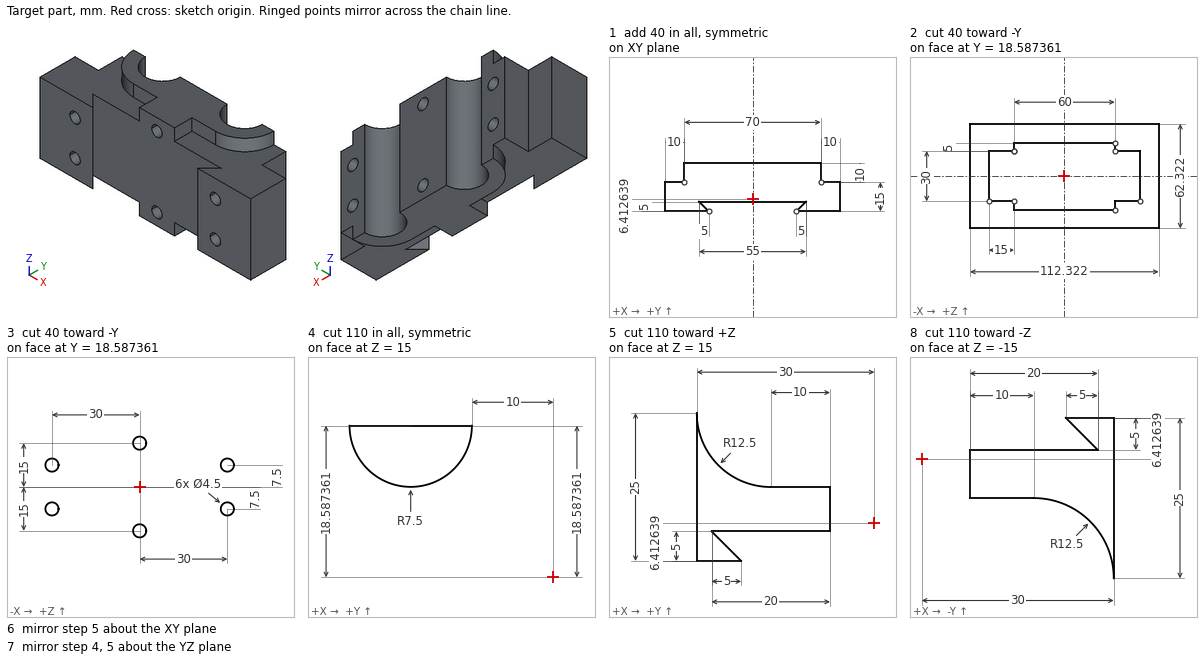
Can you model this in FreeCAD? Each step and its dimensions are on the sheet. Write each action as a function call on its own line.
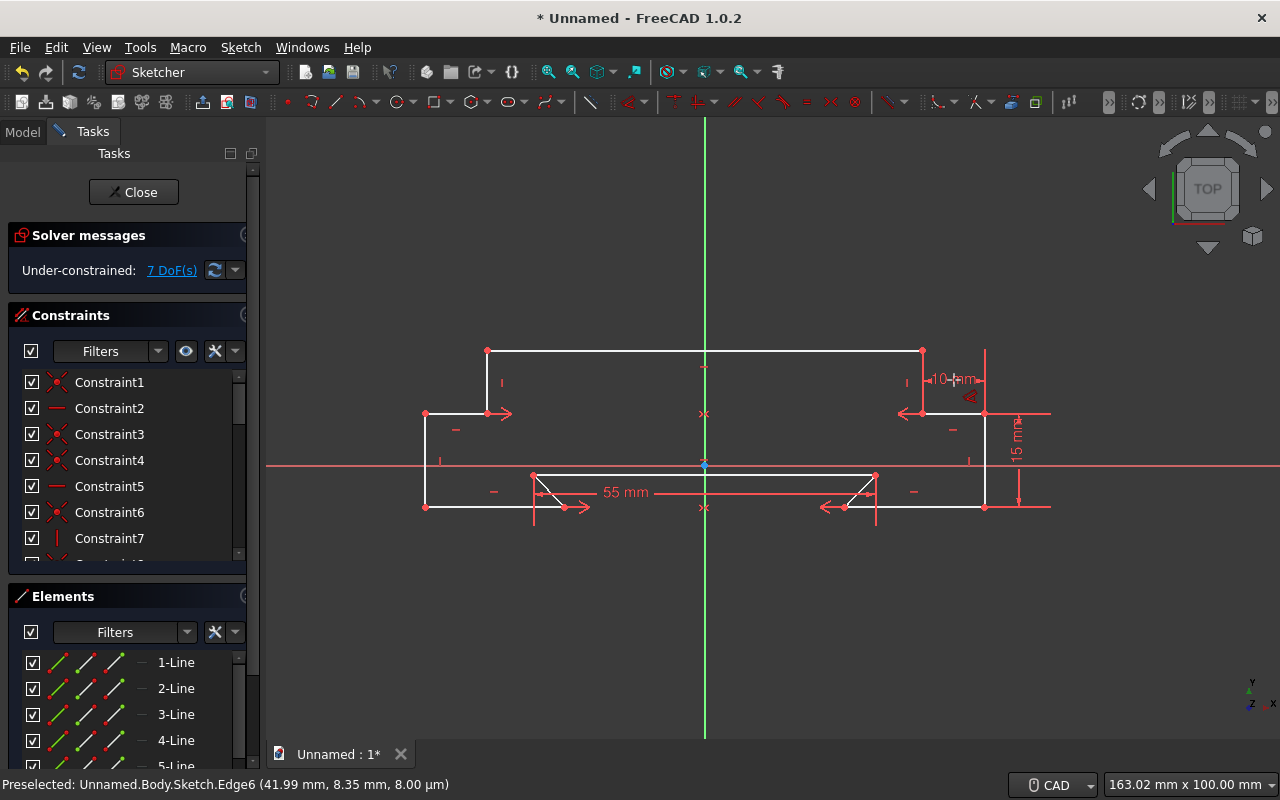
click(923, 395)
click(889, 405)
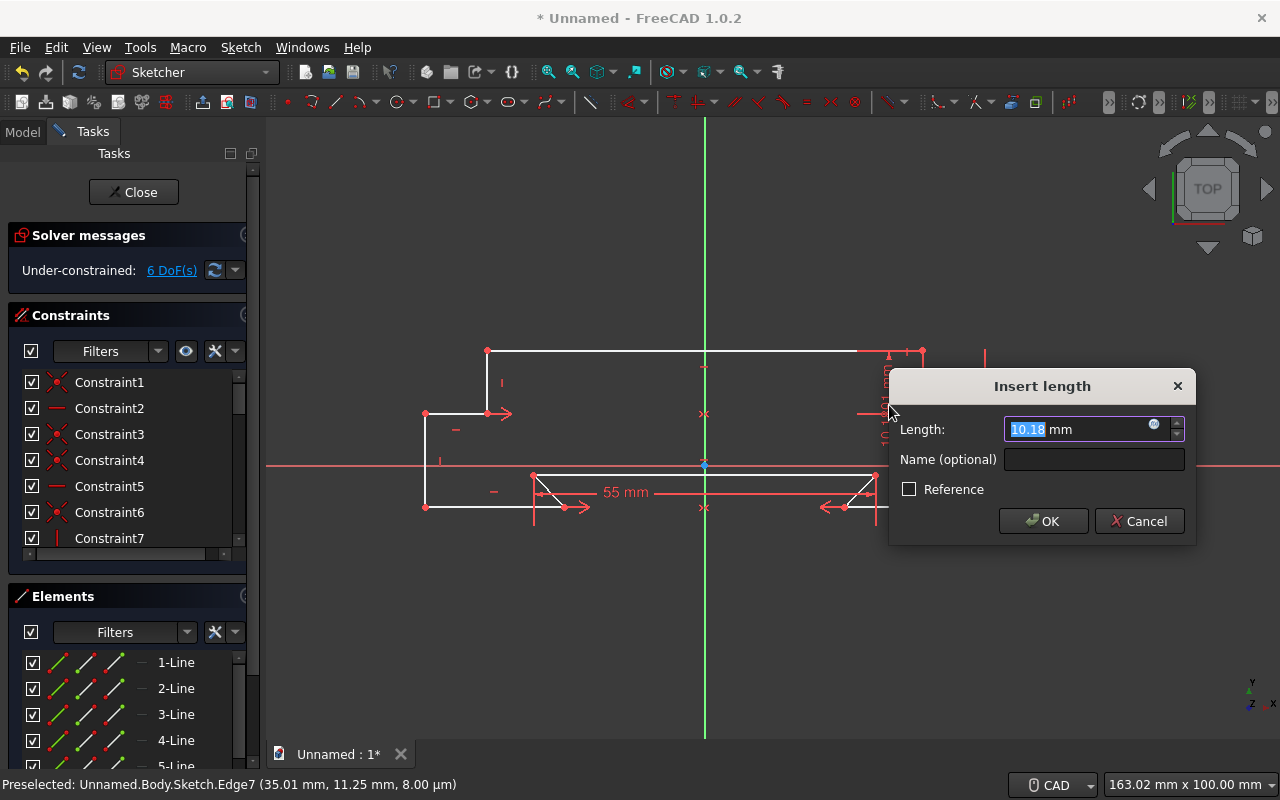
text(10)
key(Return)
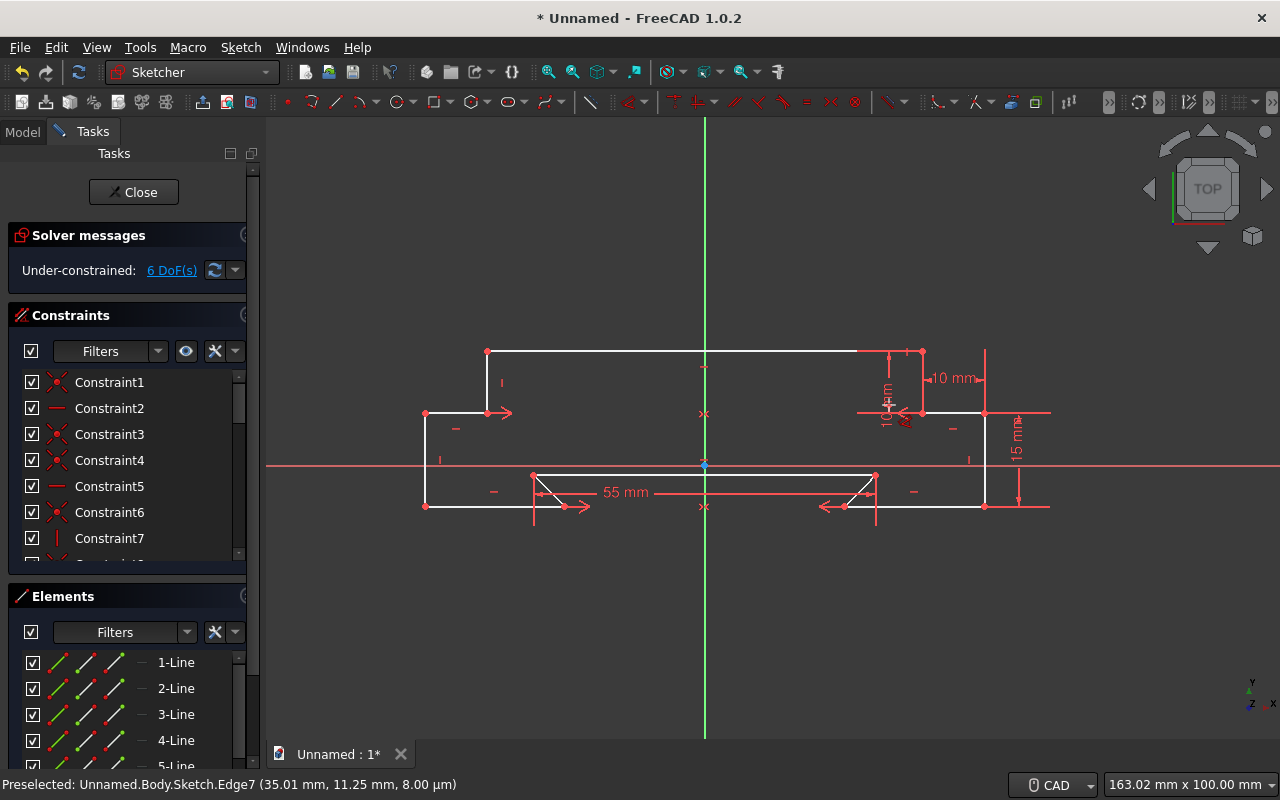
click(792, 351)
click(605, 317)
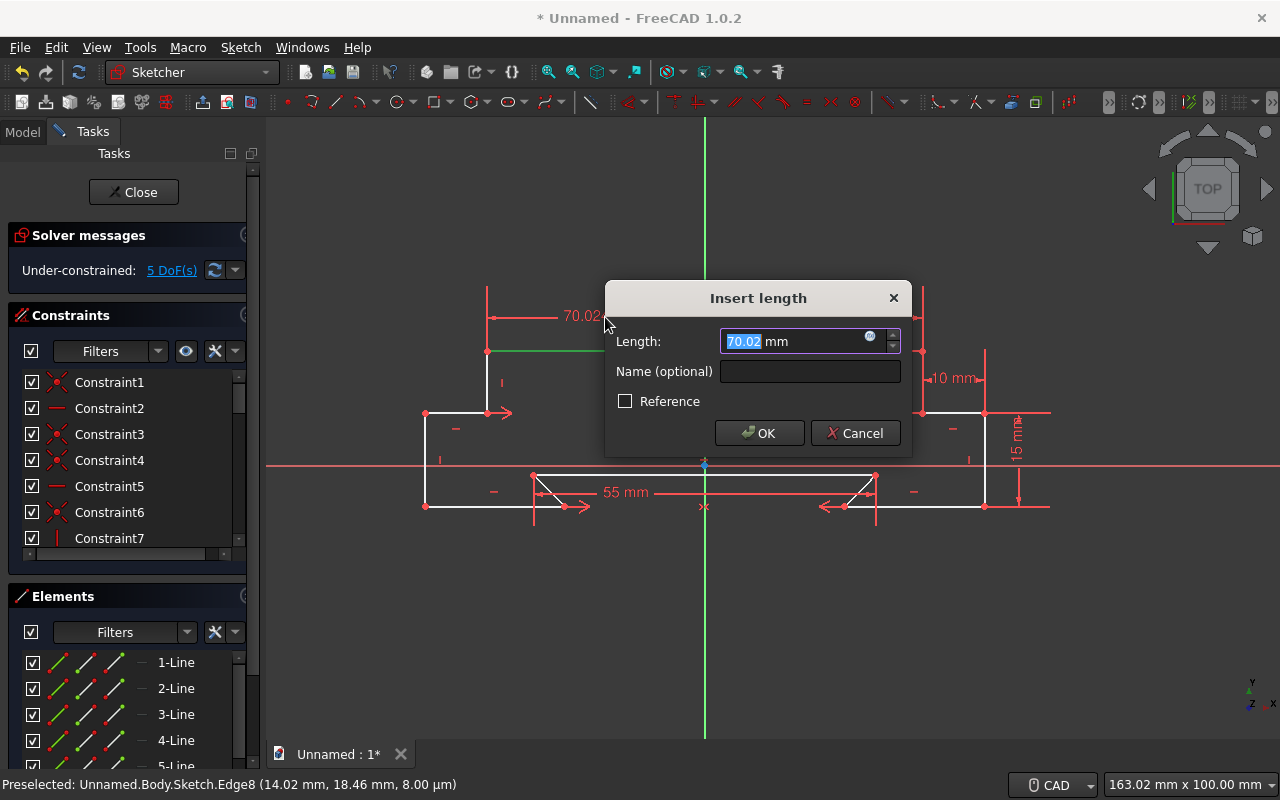
text(70)
key(Return)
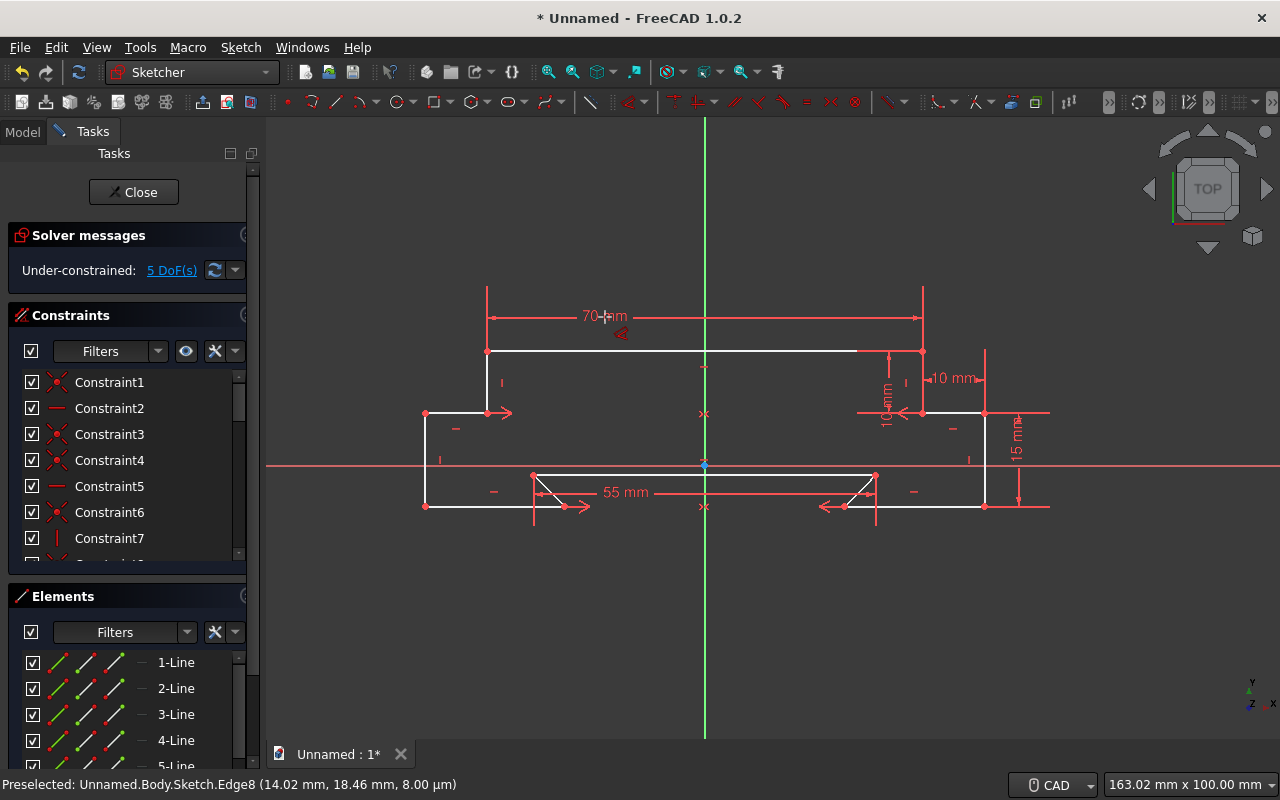
click(468, 413)
click(456, 379)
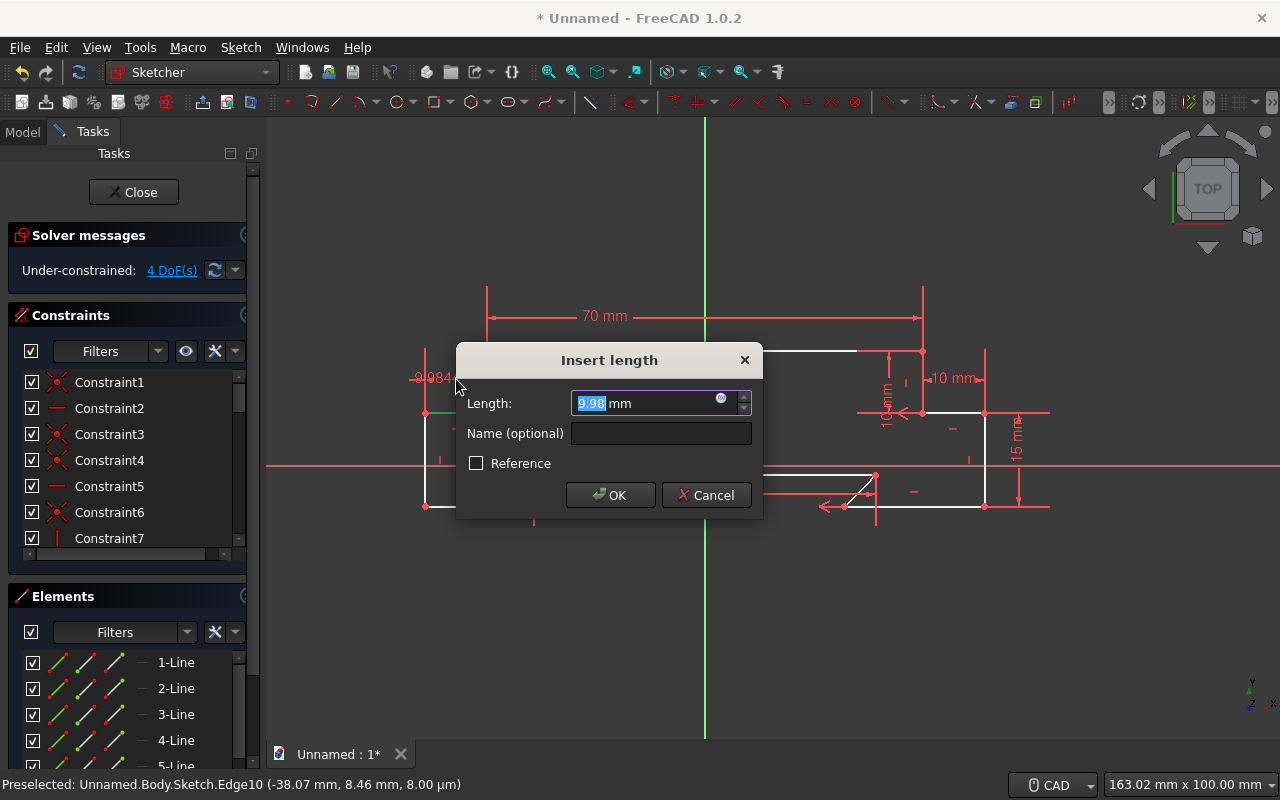
text(10)
key(Return)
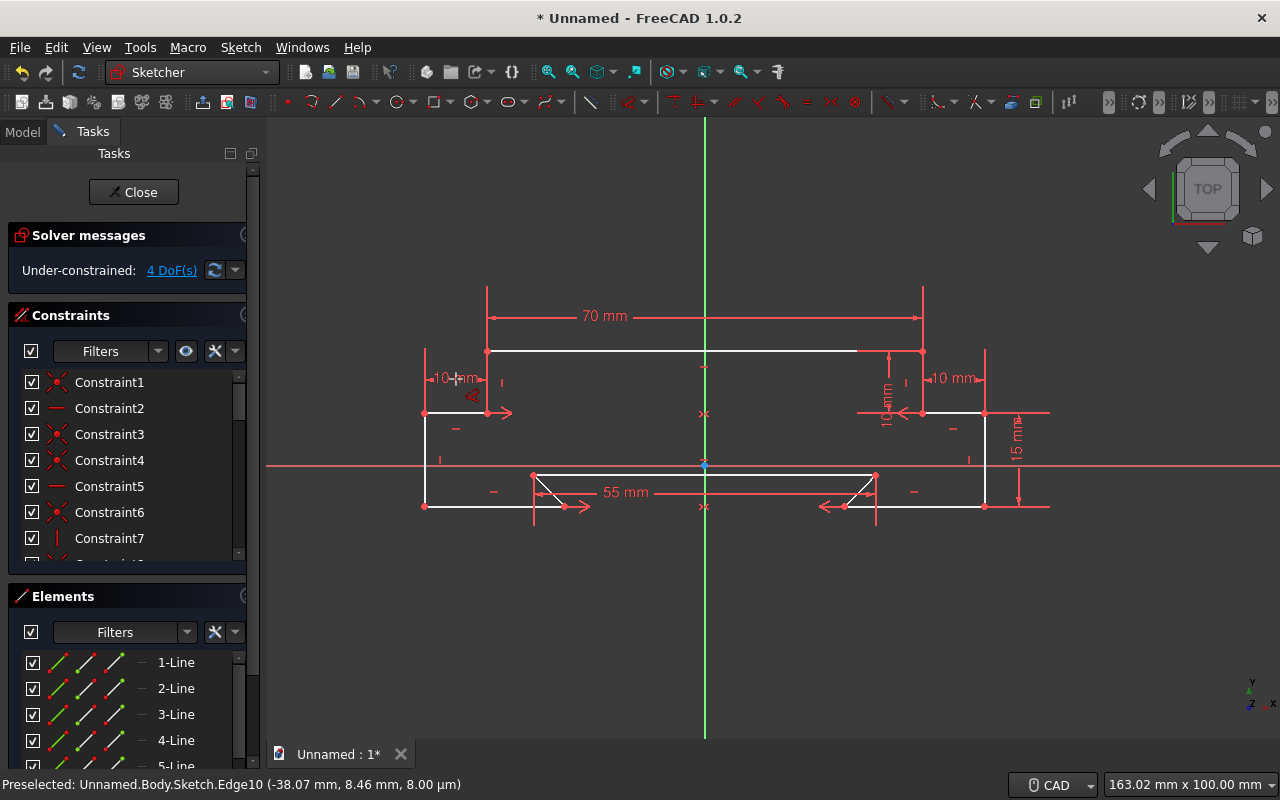
scroll(555, 497, up, 2)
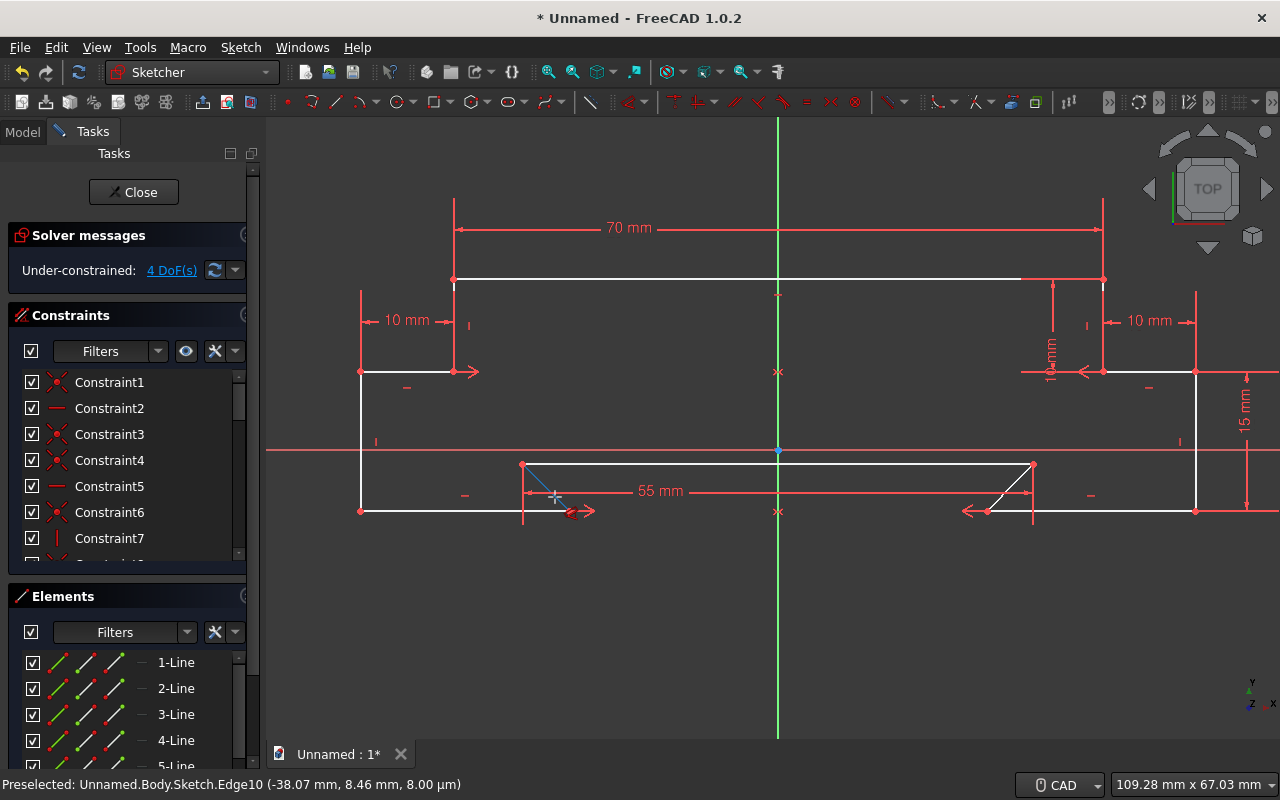
click(556, 497)
click(546, 545)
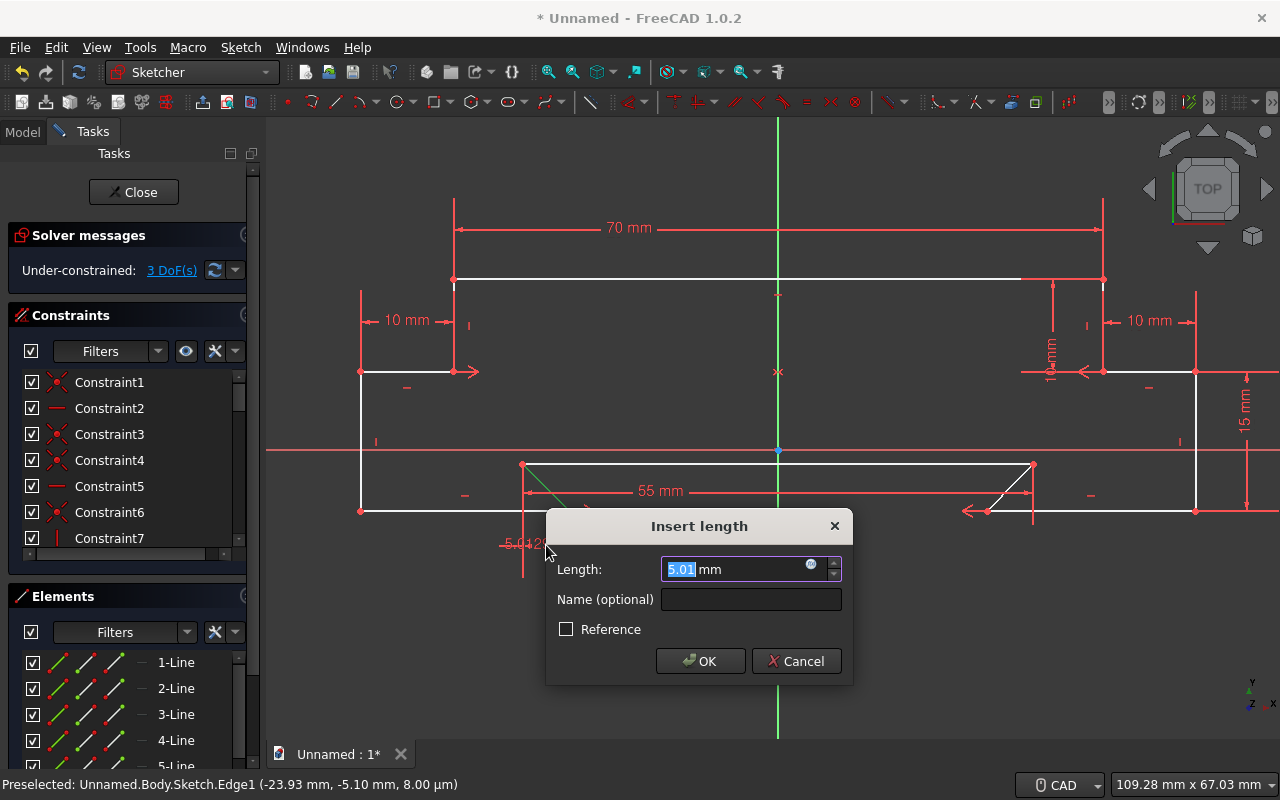
text(5)
key(Return)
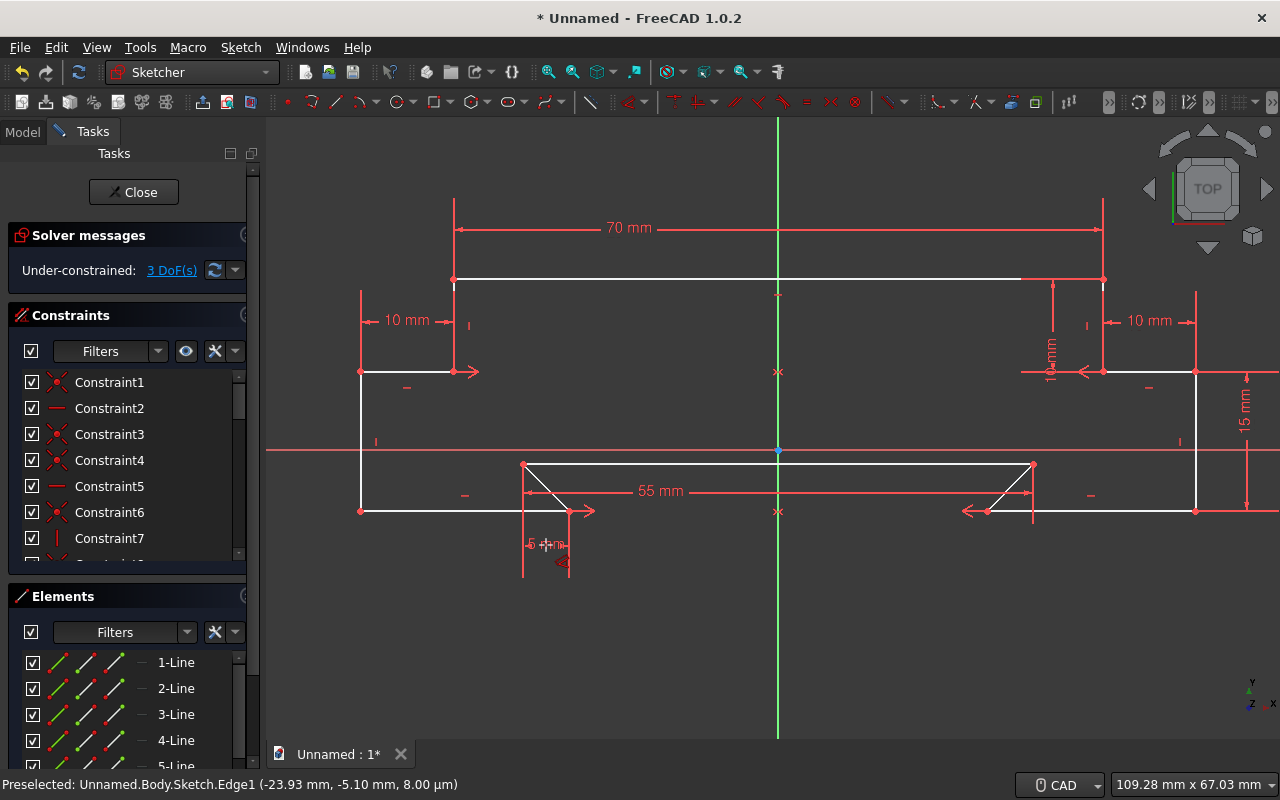
click(556, 497)
click(489, 488)